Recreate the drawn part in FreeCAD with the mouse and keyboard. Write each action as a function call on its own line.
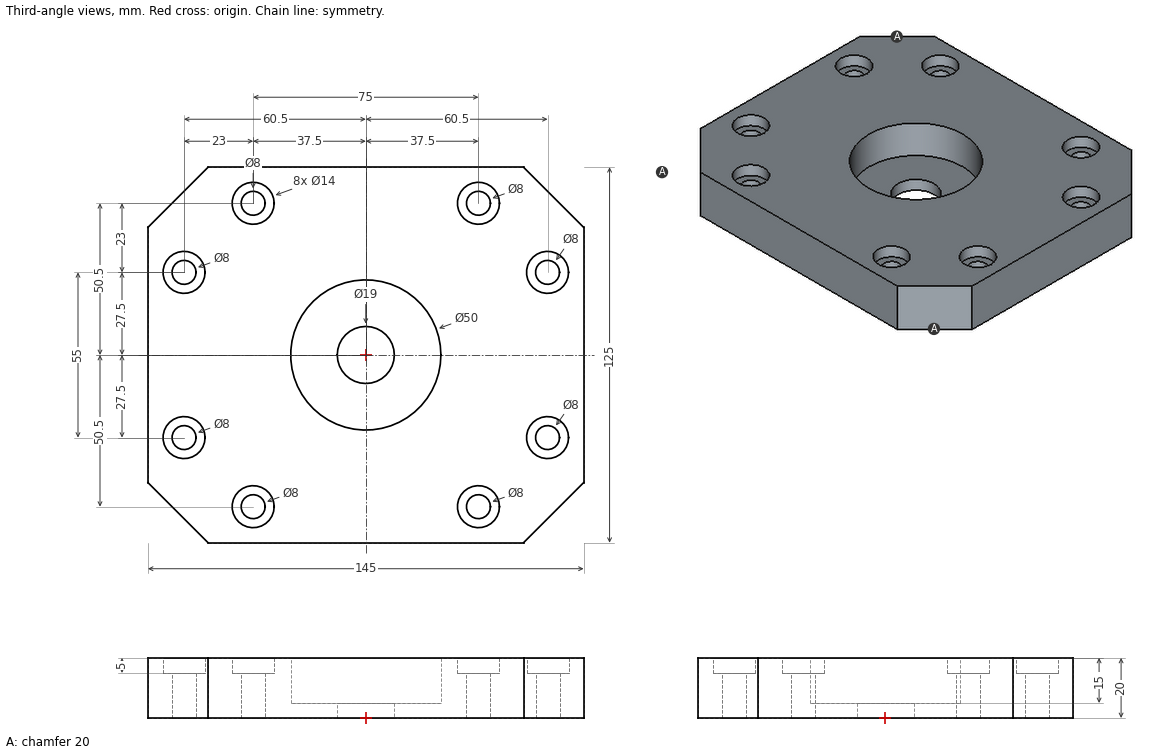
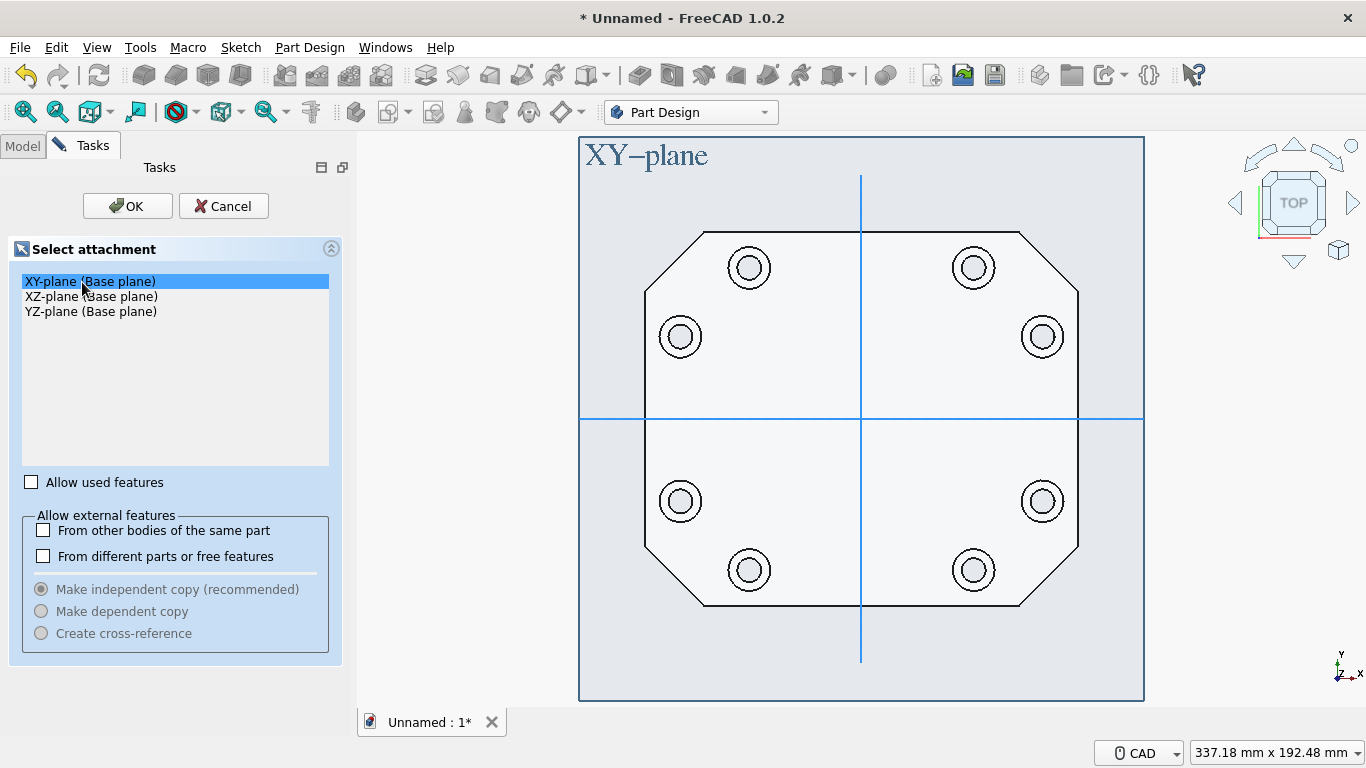
click(128, 206)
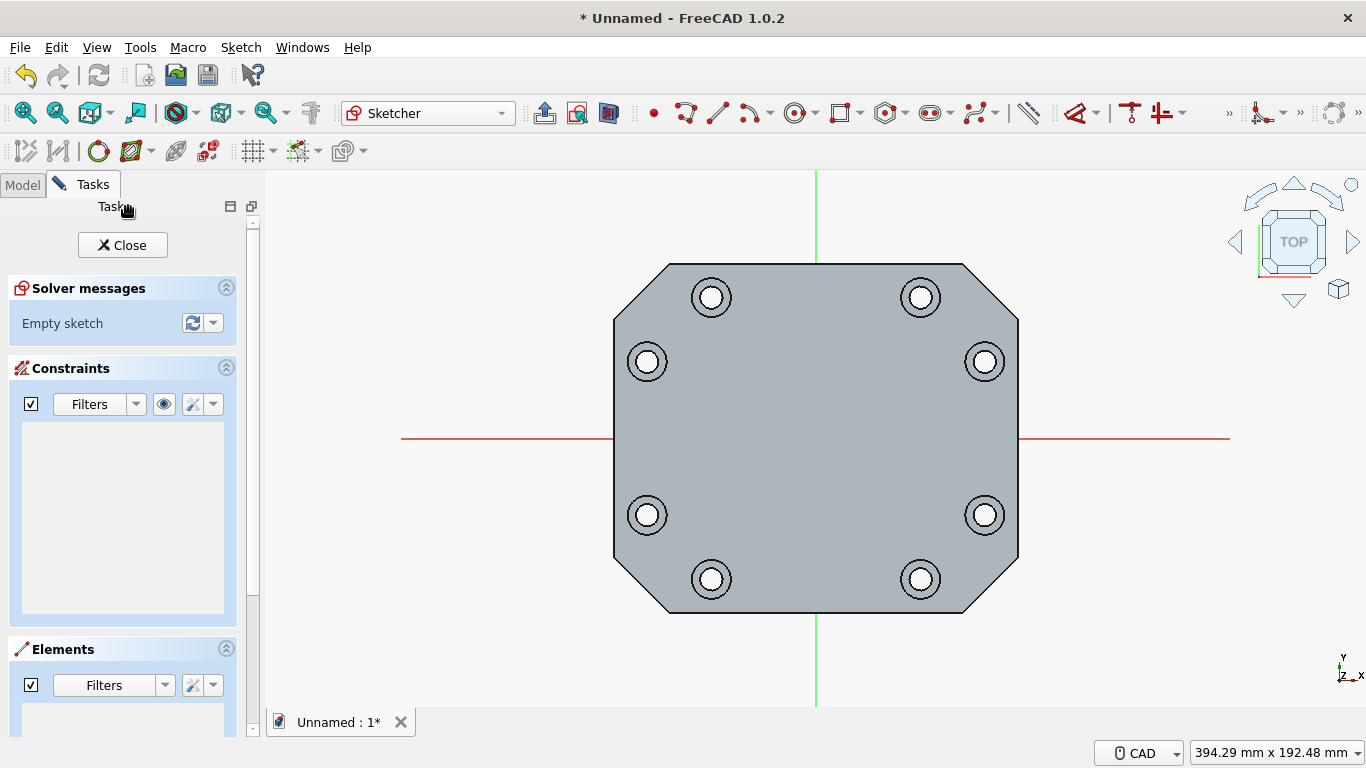
click(610, 114)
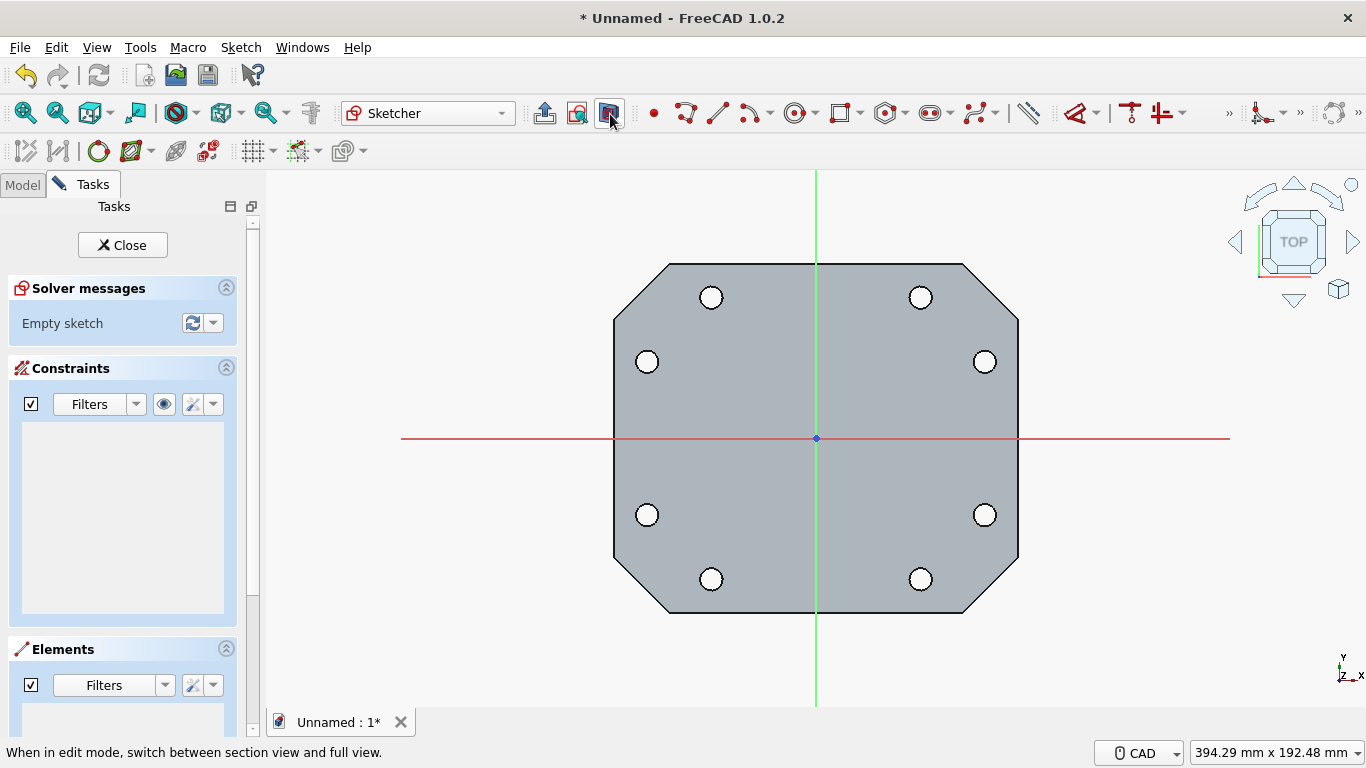
scroll(830, 438, up, 9)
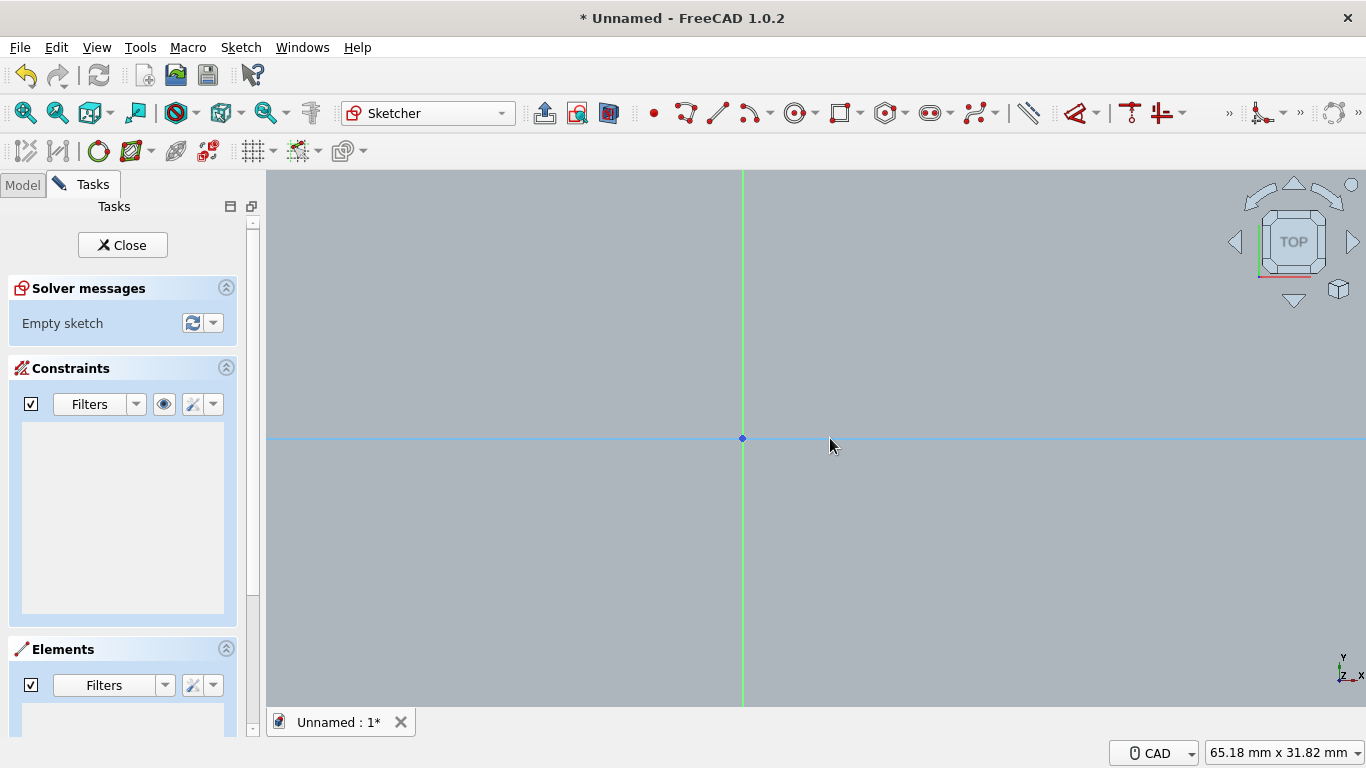
click(796, 114)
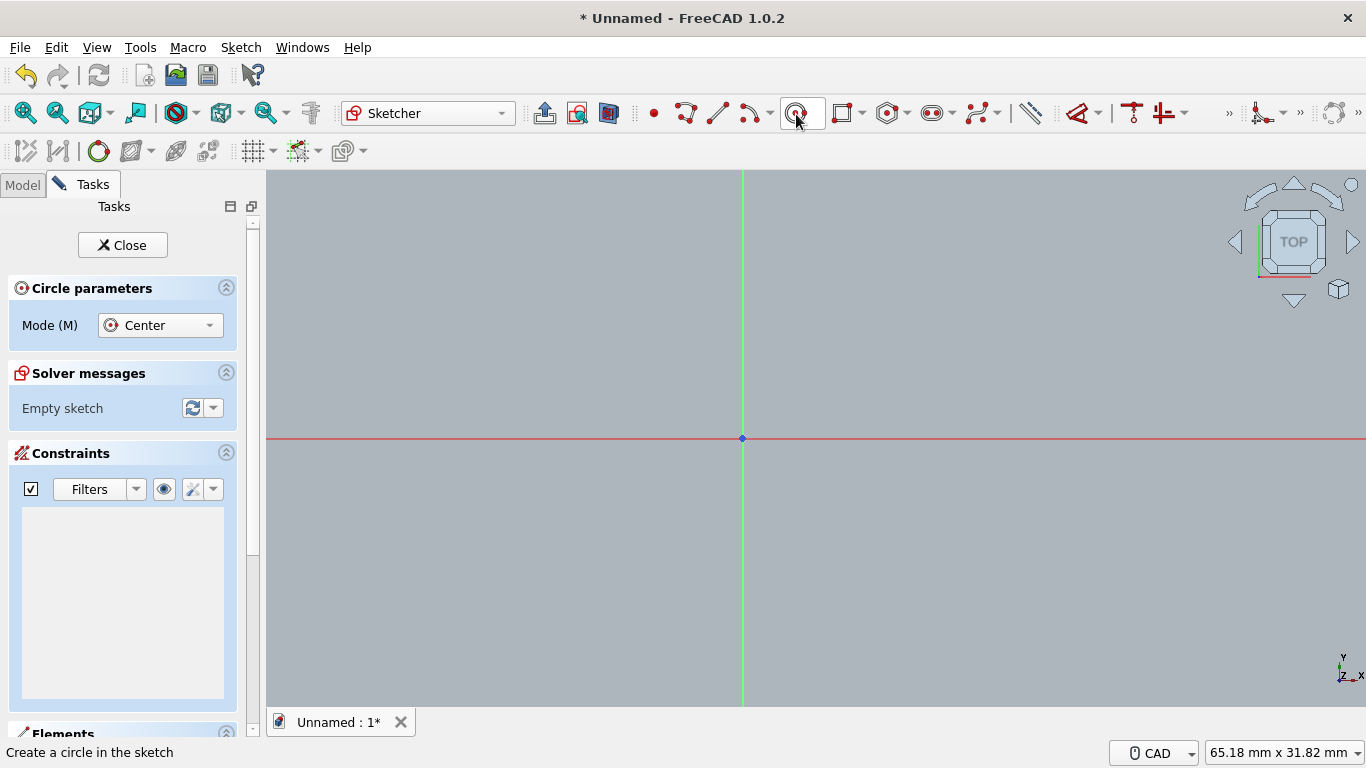
click(743, 438)
click(856, 325)
key(Escape)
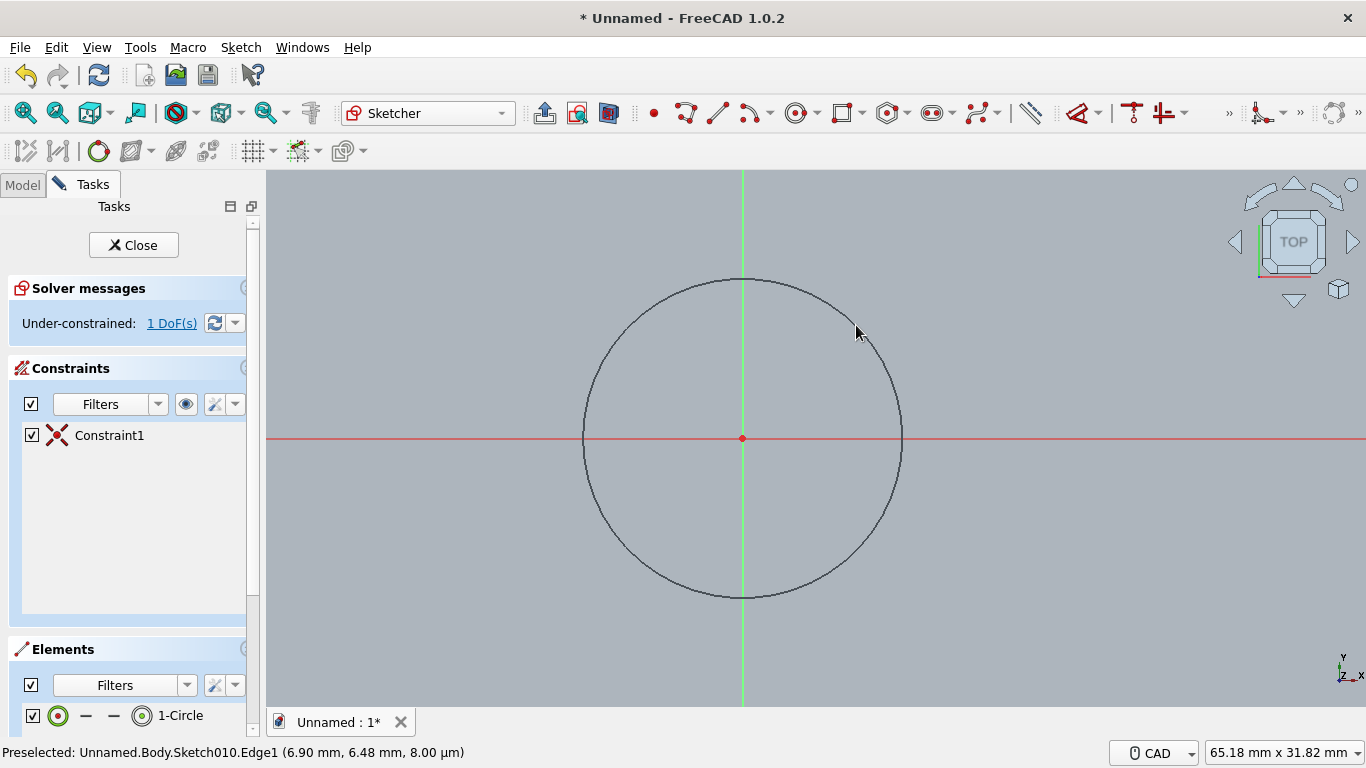
click(1078, 114)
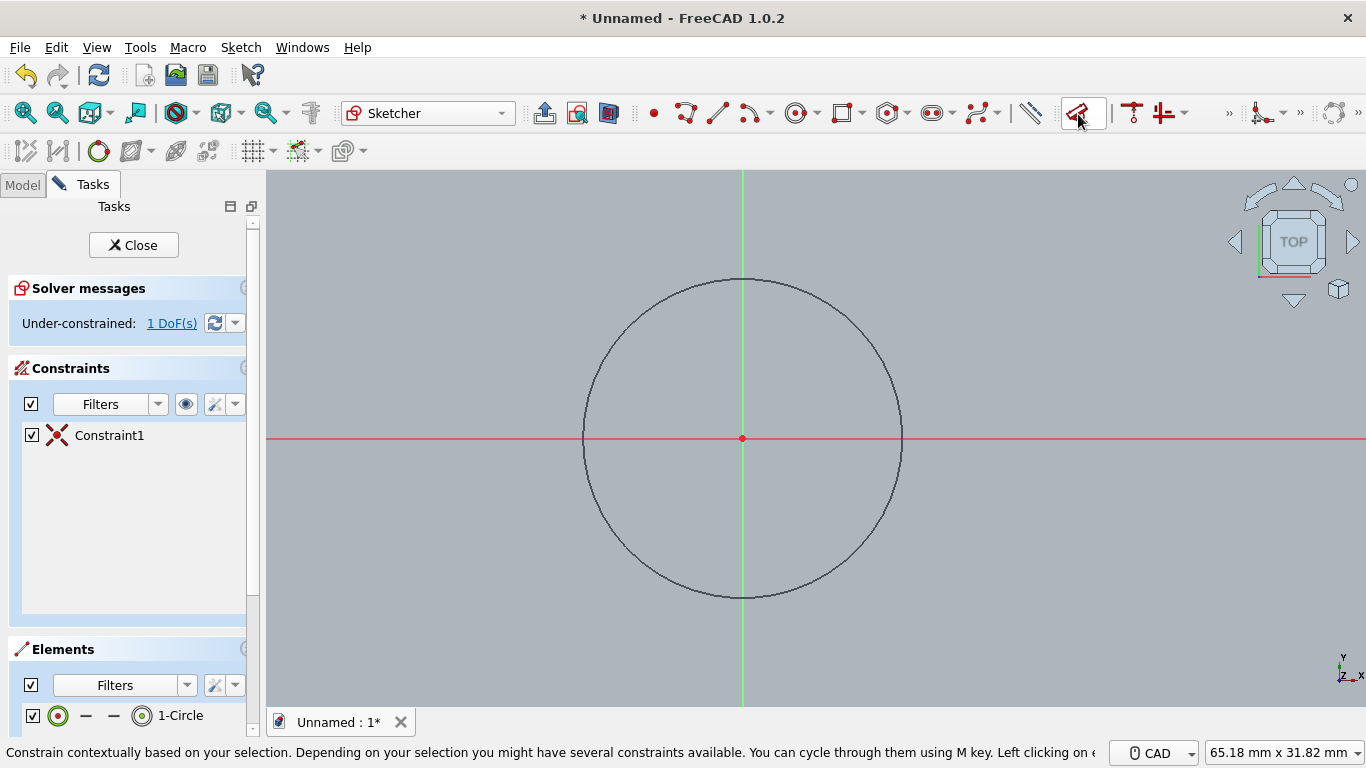
click(855, 325)
click(878, 302)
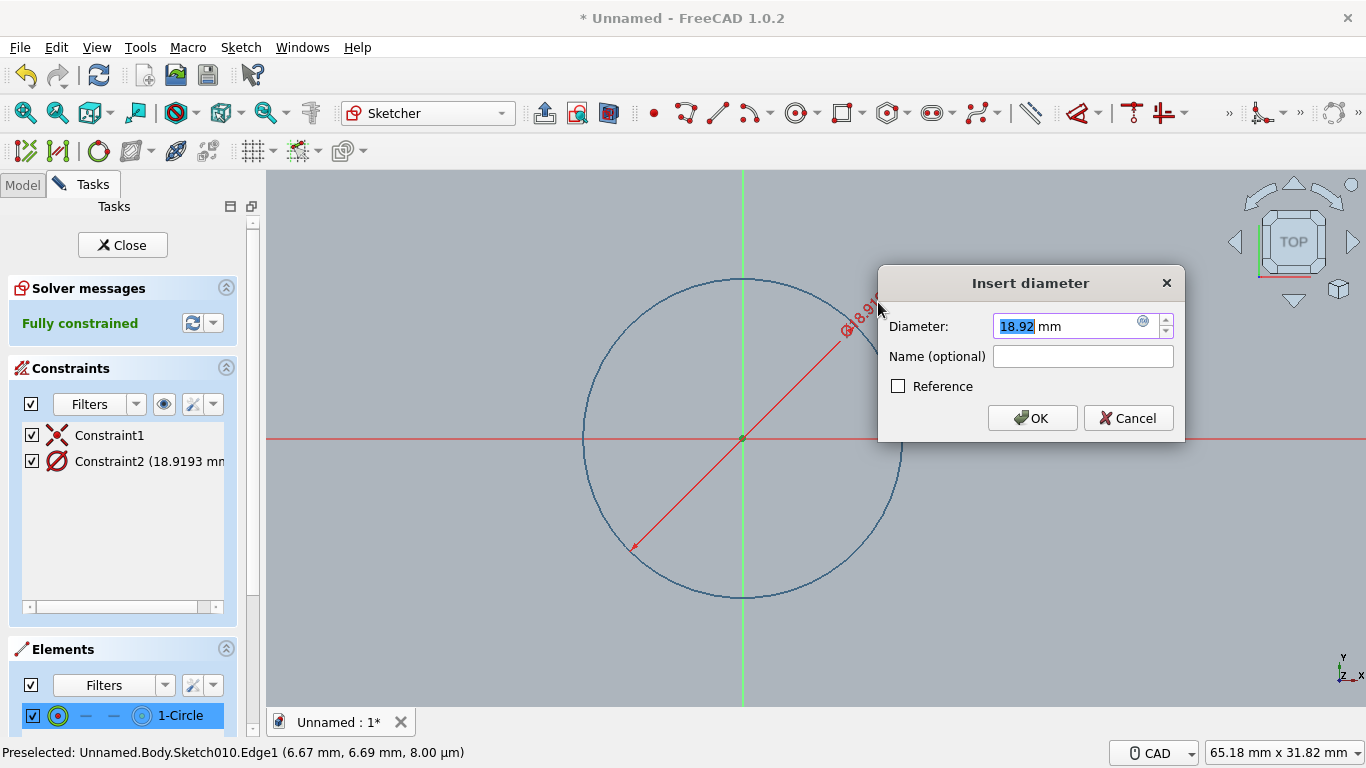
text(19)
key(Return)
key(Escape)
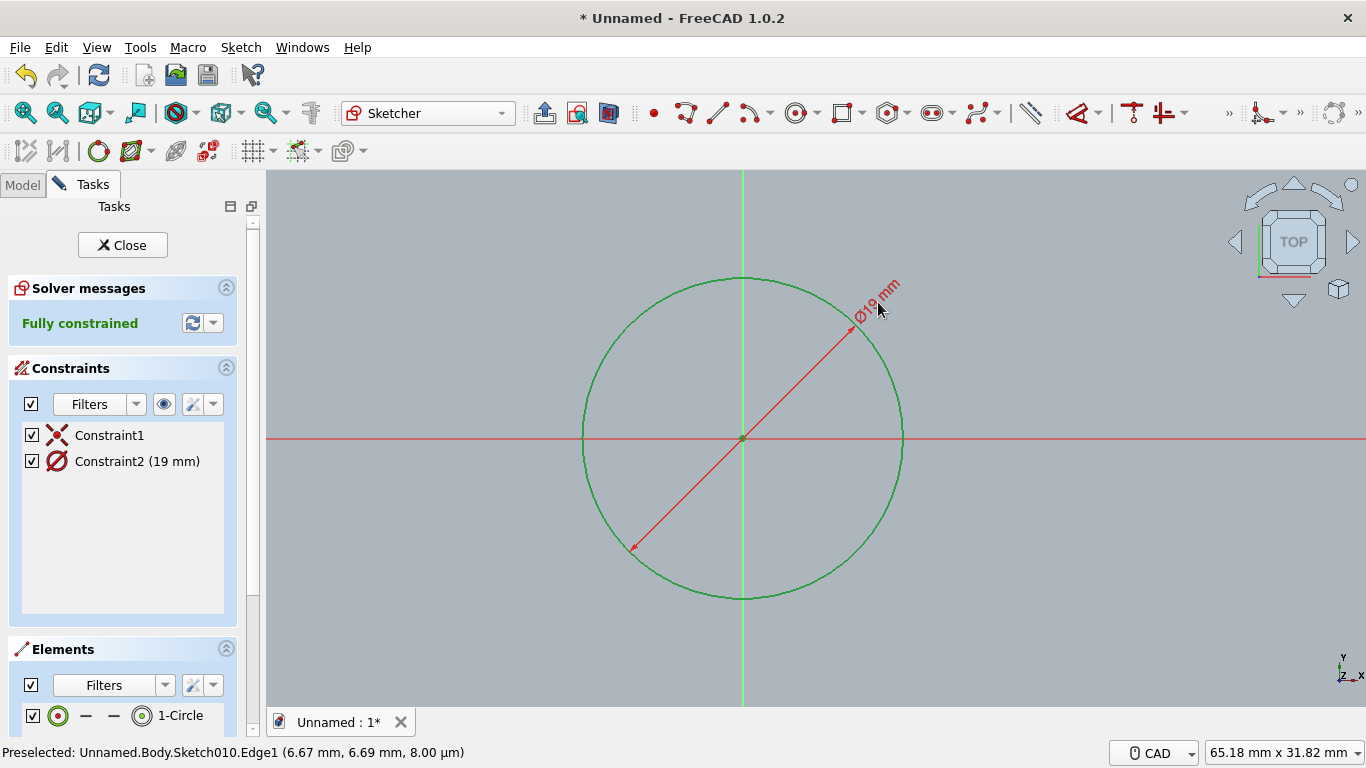
click(123, 245)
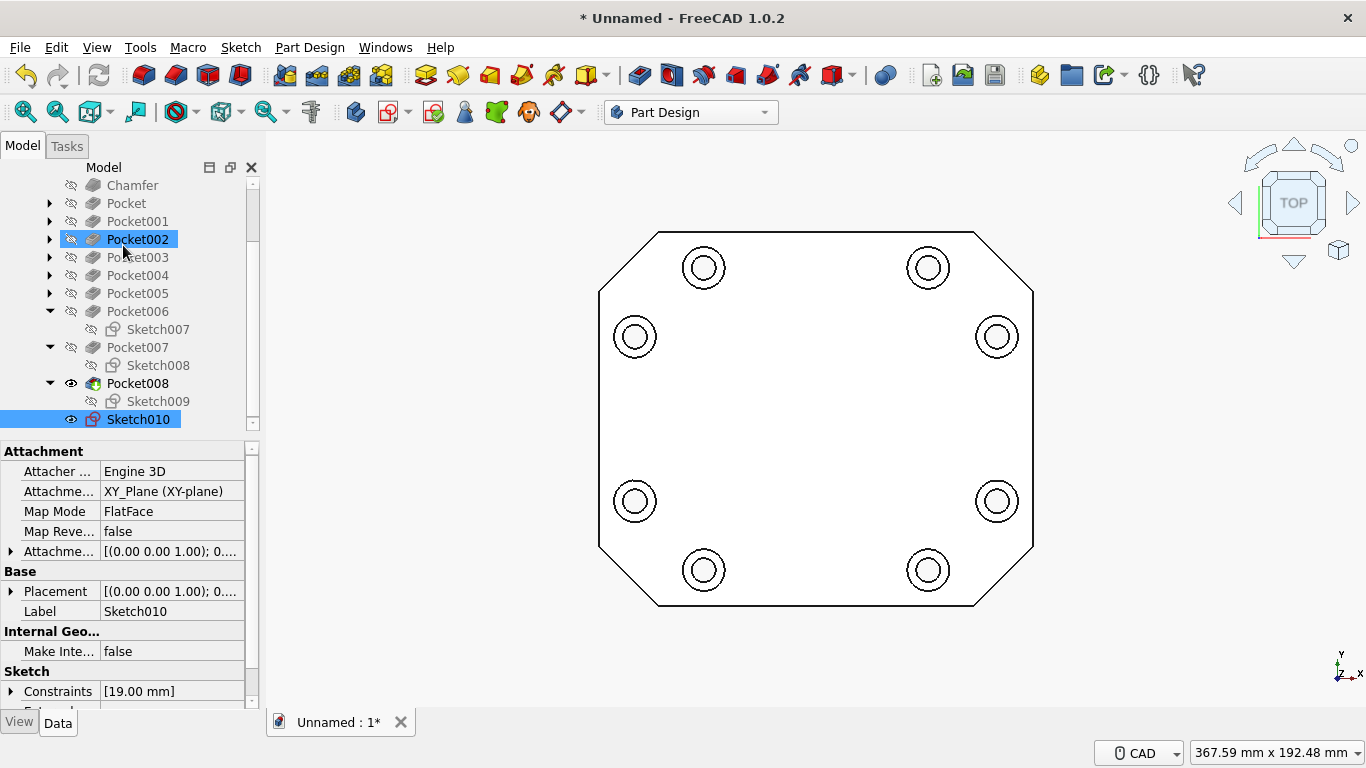
click(640, 76)